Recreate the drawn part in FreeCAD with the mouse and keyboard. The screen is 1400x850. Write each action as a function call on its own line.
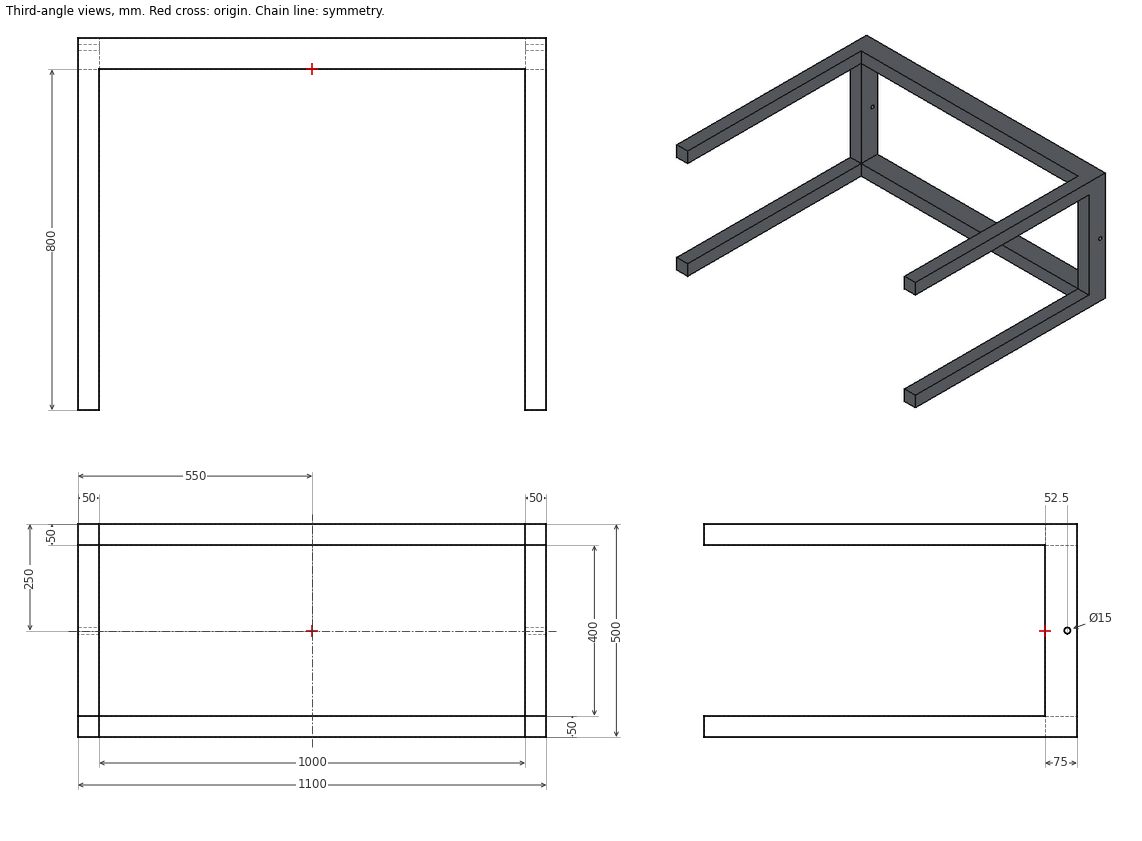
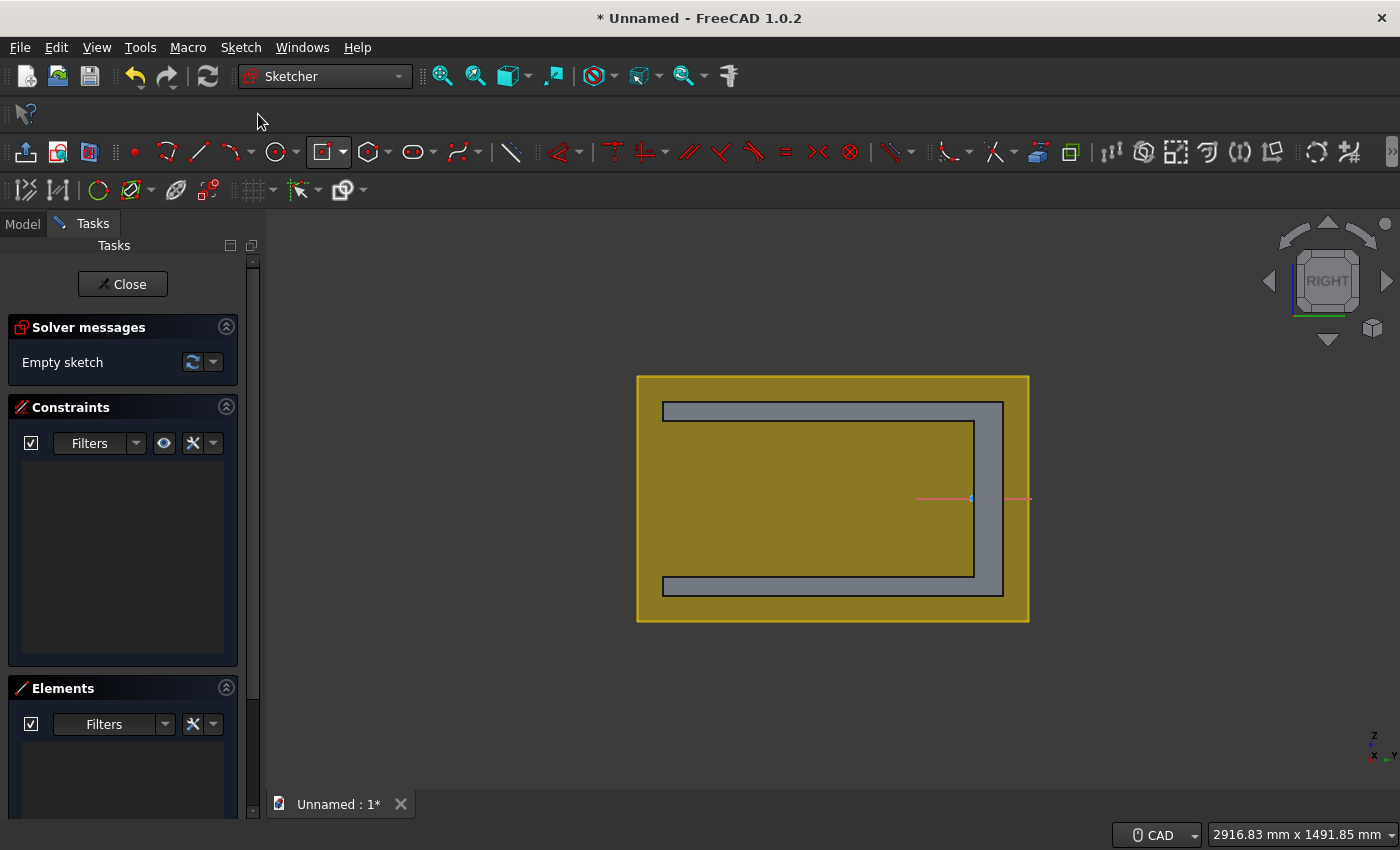
click(90, 152)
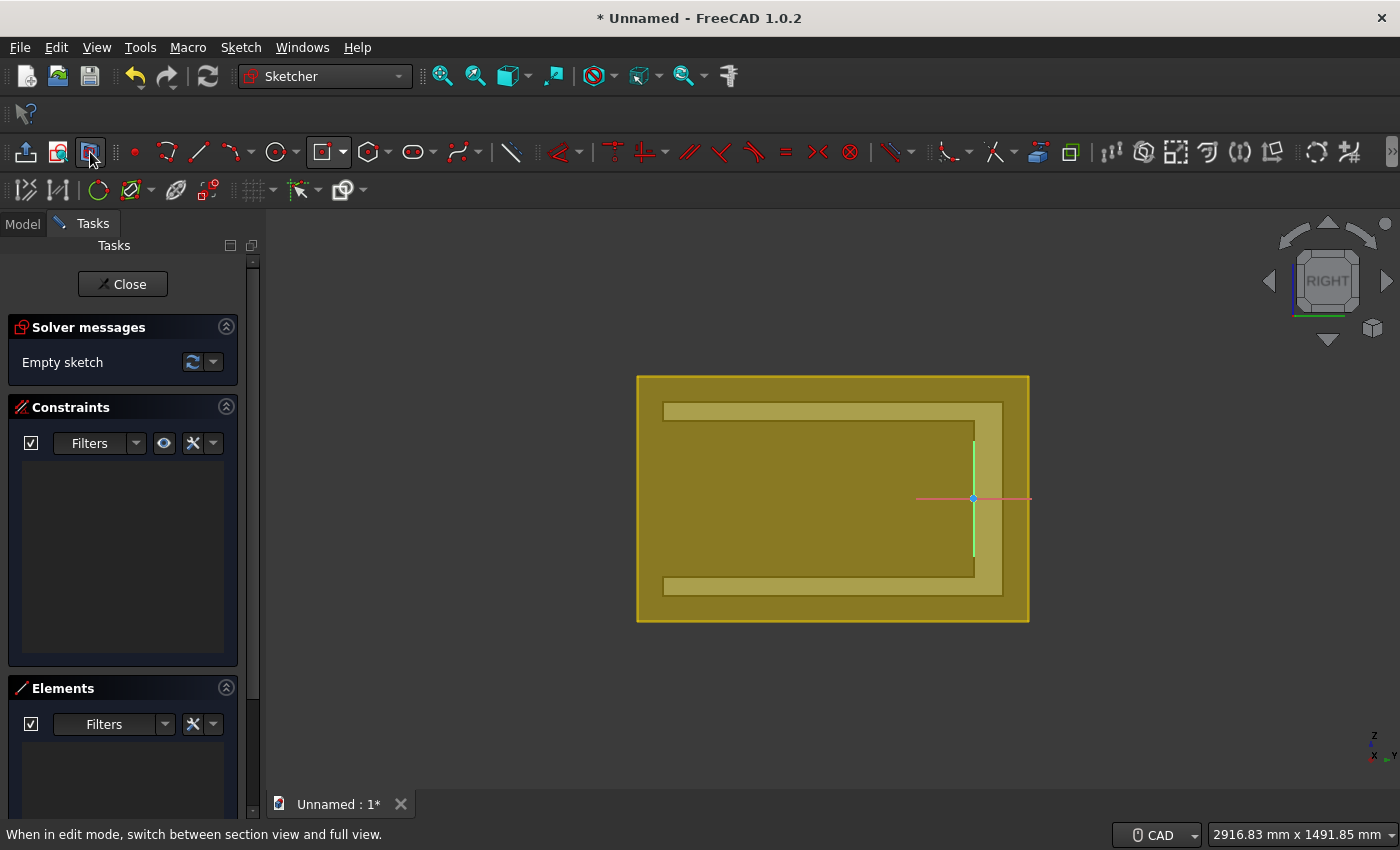
scroll(1006, 499, up, 15)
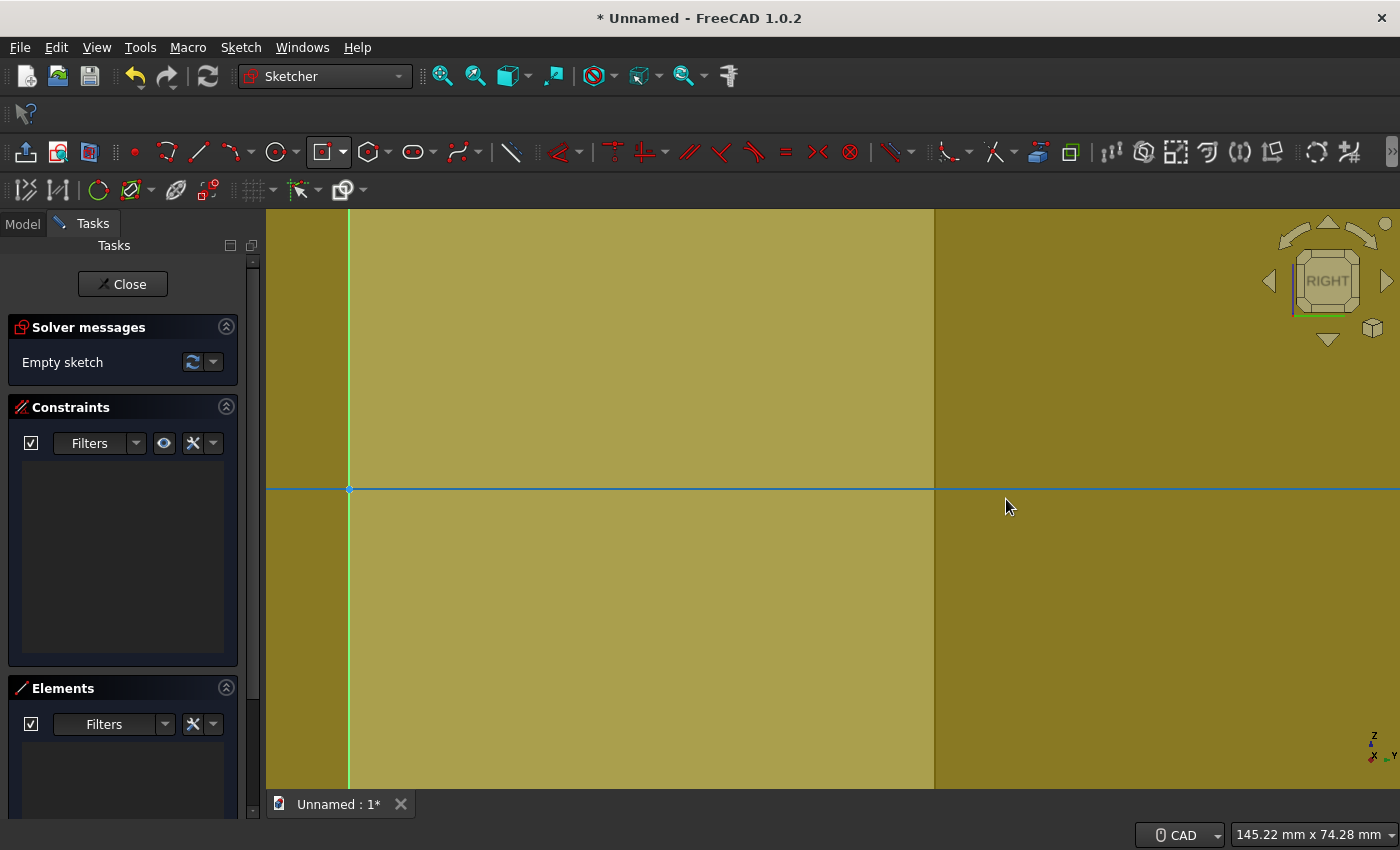
scroll(757, 485, up, 6)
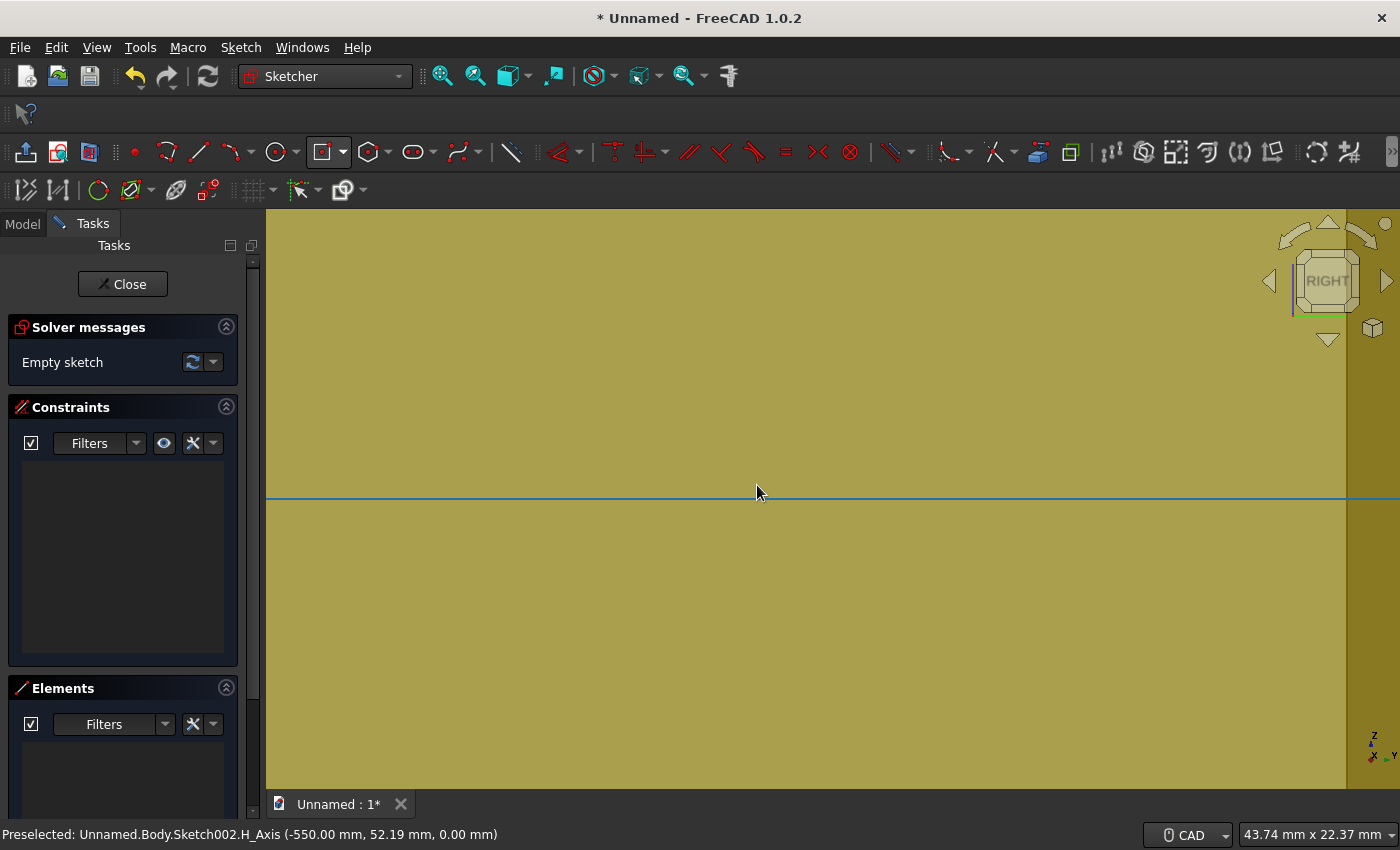
click(276, 152)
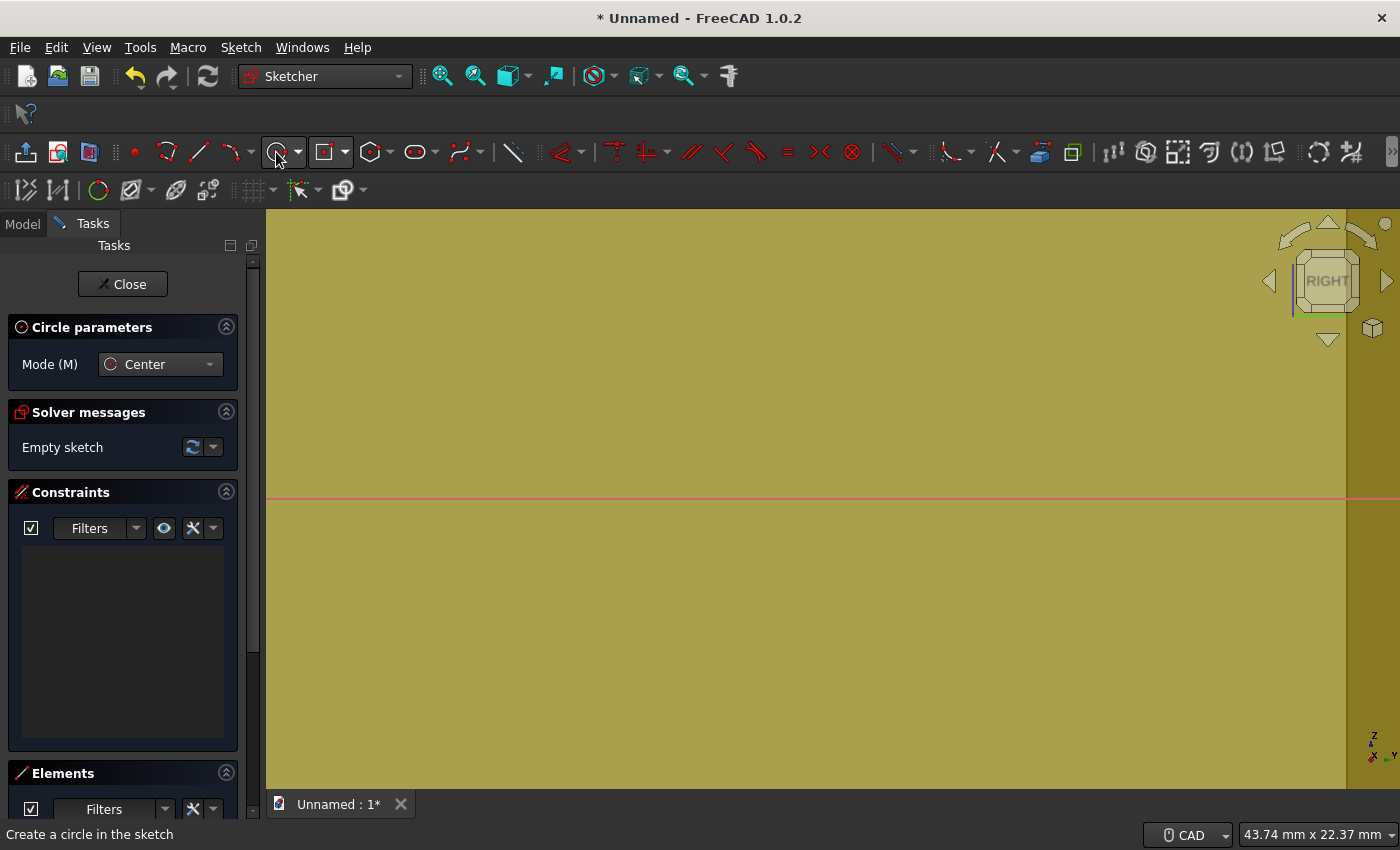
click(764, 499)
move(901, 361)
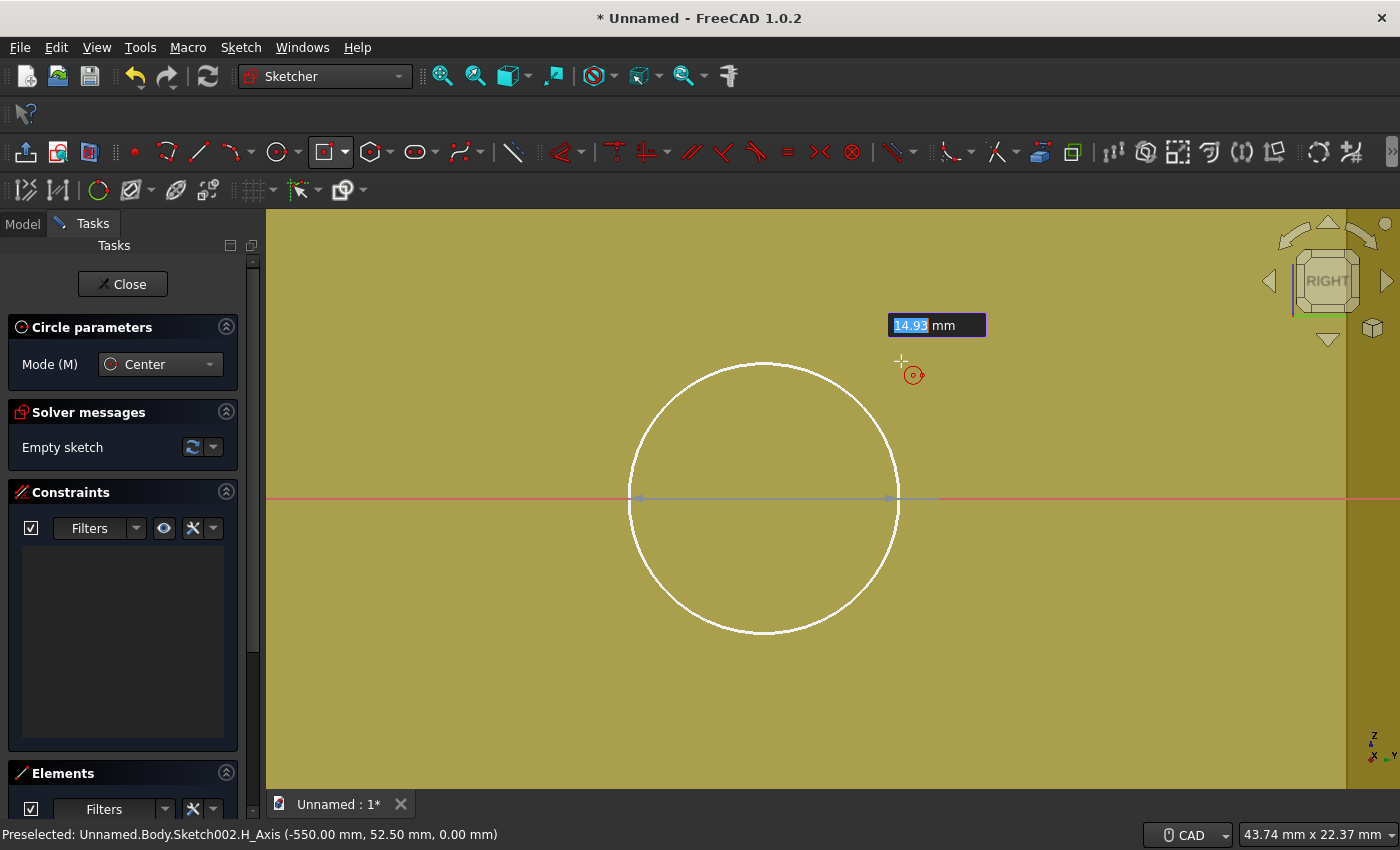
text(15)
key(Return)
key(Escape)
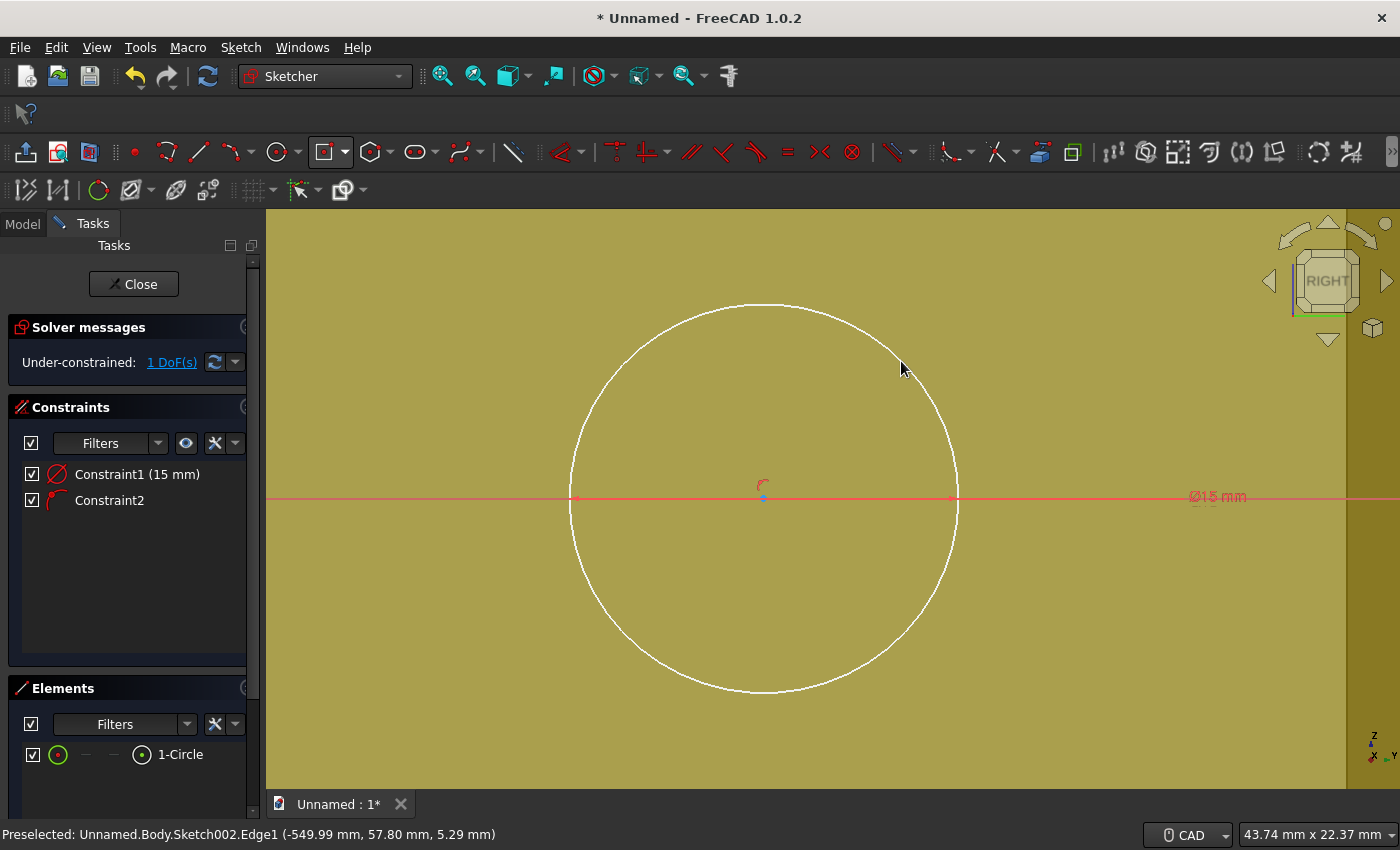
click(560, 152)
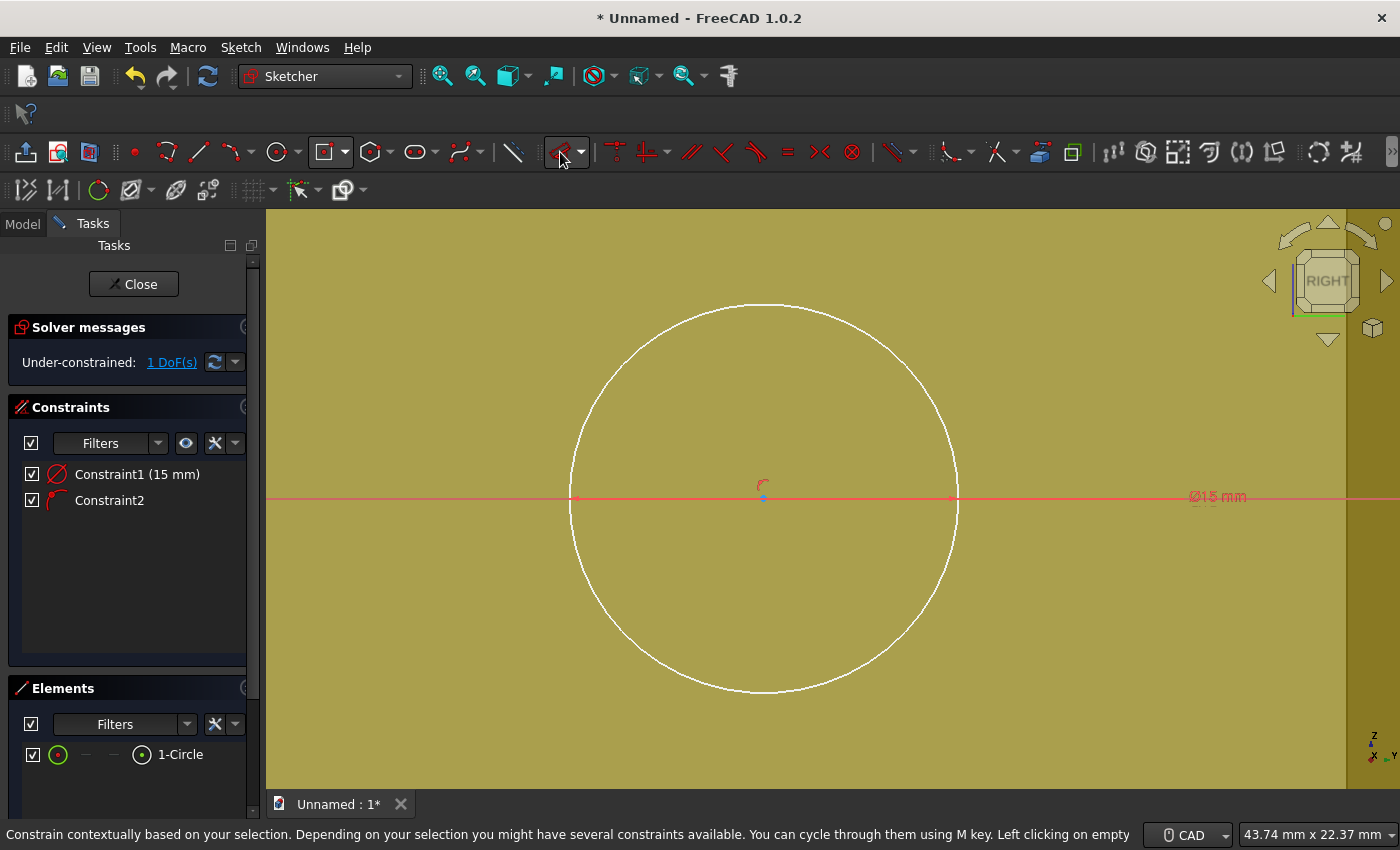
click(764, 499)
click(529, 533)